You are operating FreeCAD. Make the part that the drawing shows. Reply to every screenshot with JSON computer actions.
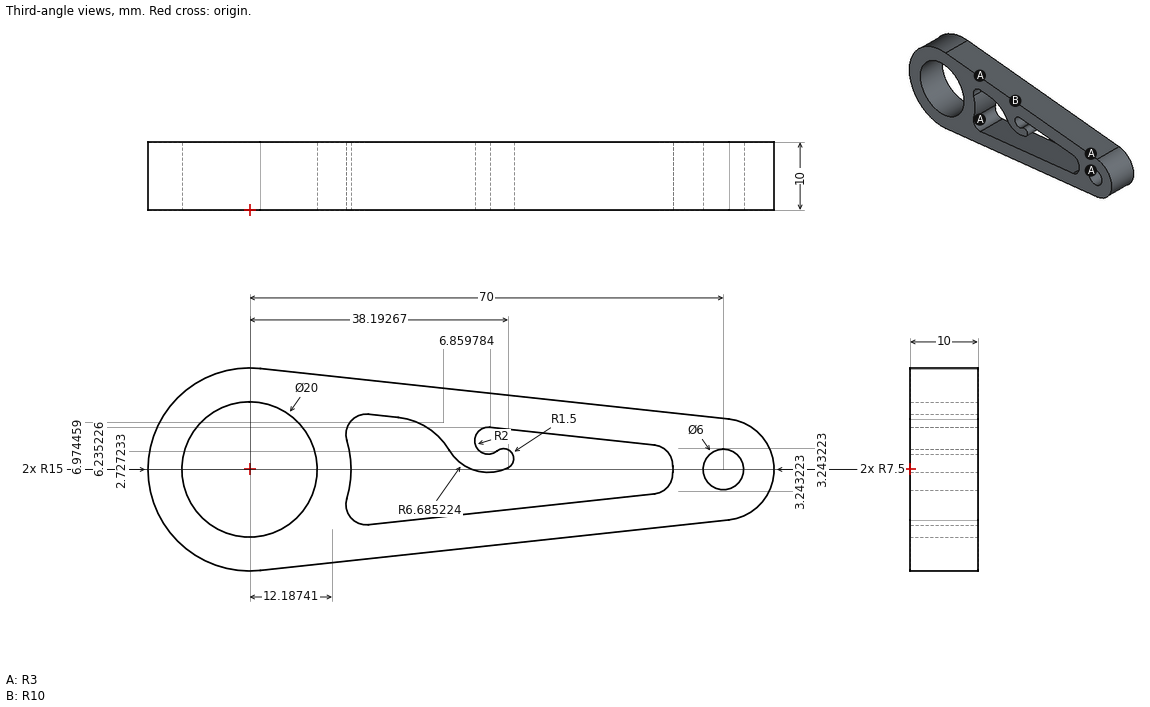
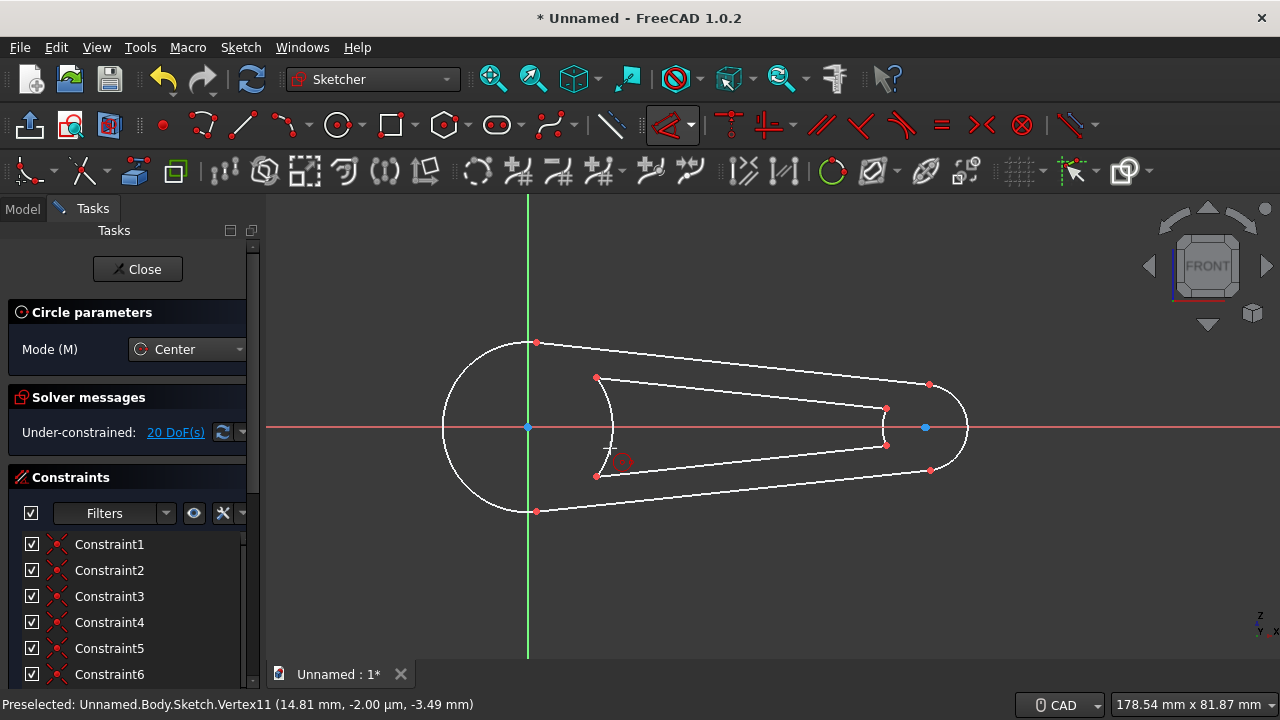
{"action": "scroll", "coordinate": [925, 427], "scroll_direction": "up", "scroll_amount": 2}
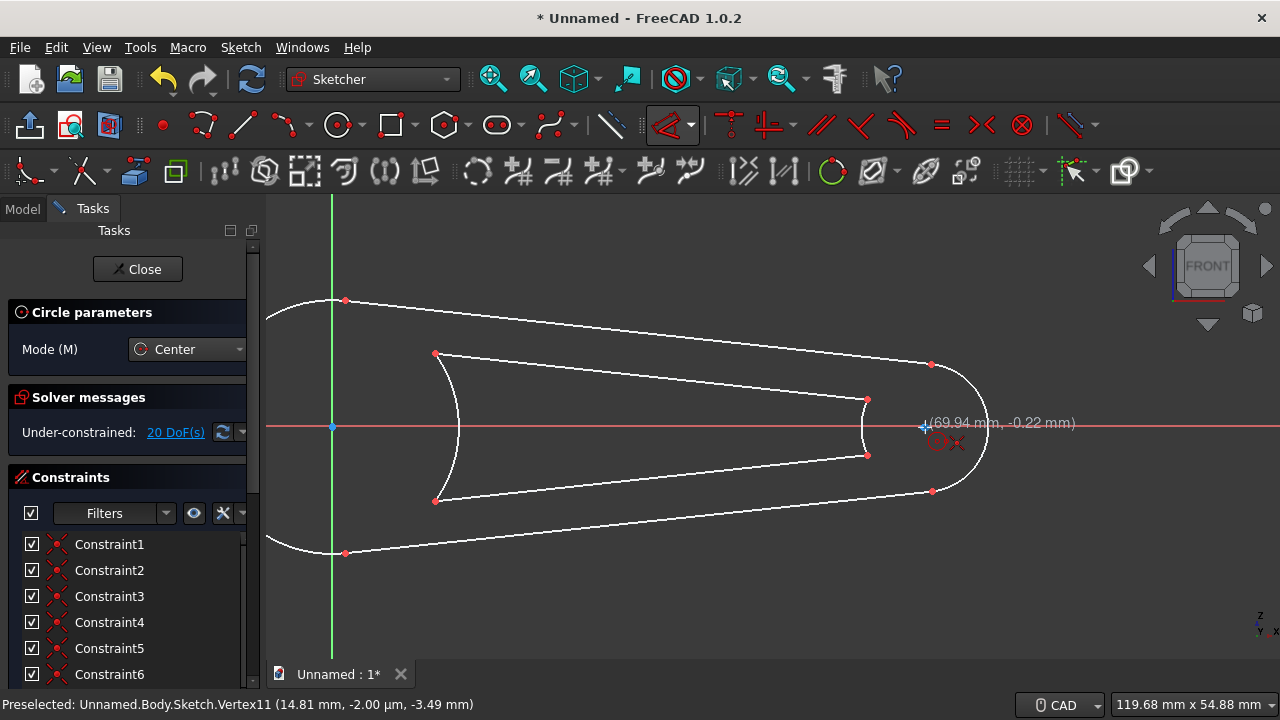
{"action": "left_click", "coordinate": [925, 426]}
{"action": "mouse_move", "coordinate": [943, 408]}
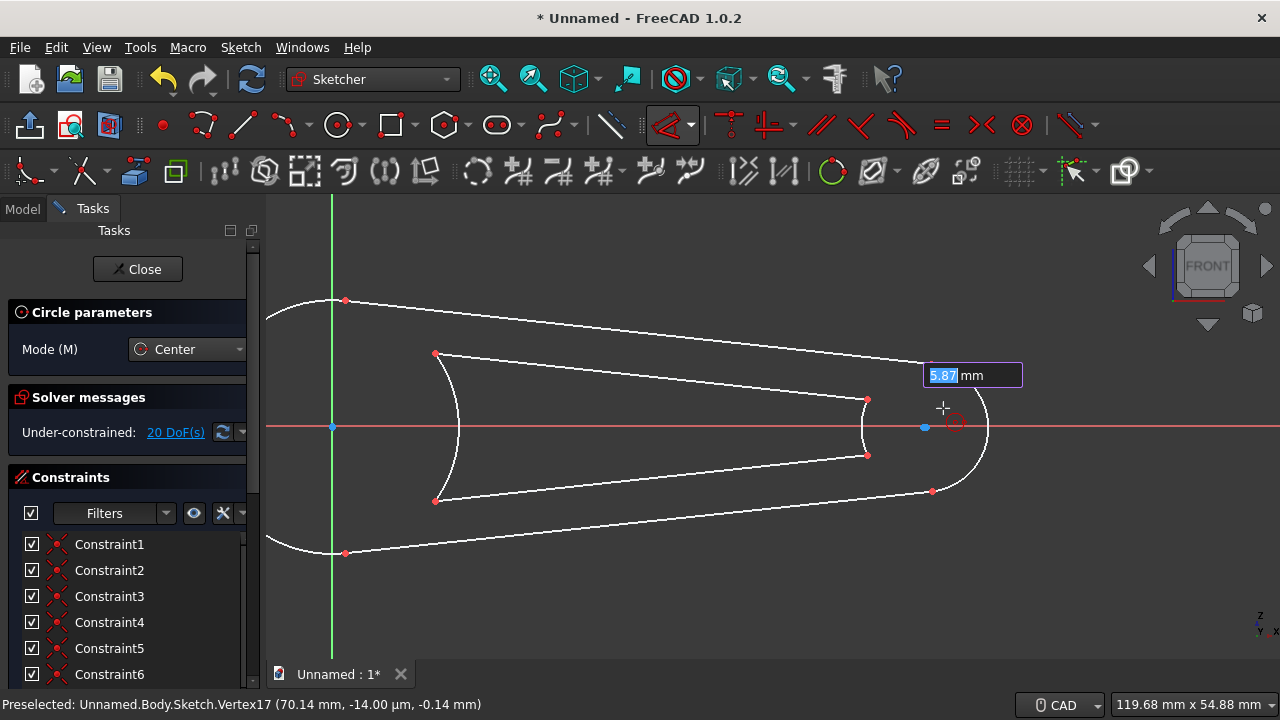
{"action": "type", "text": "6"}
{"action": "key", "text": "Return"}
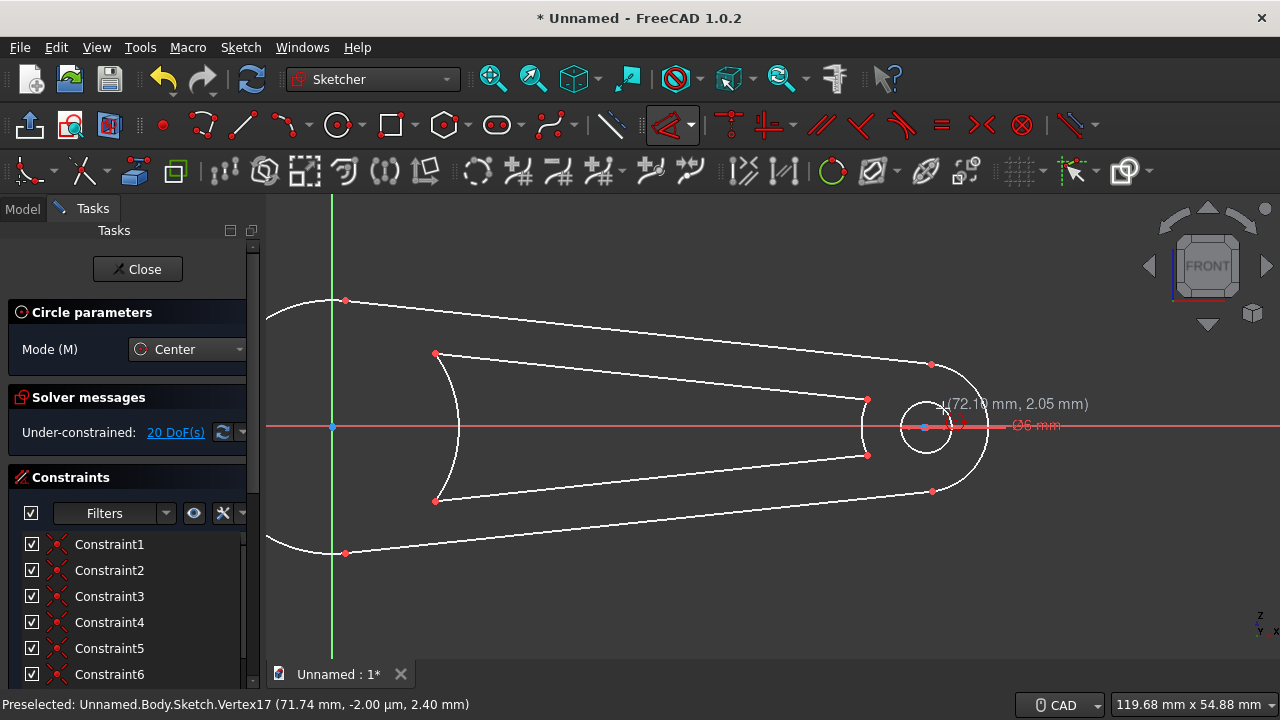
{"action": "left_click", "coordinate": [332, 426]}
{"action": "mouse_move", "coordinate": [392, 366]}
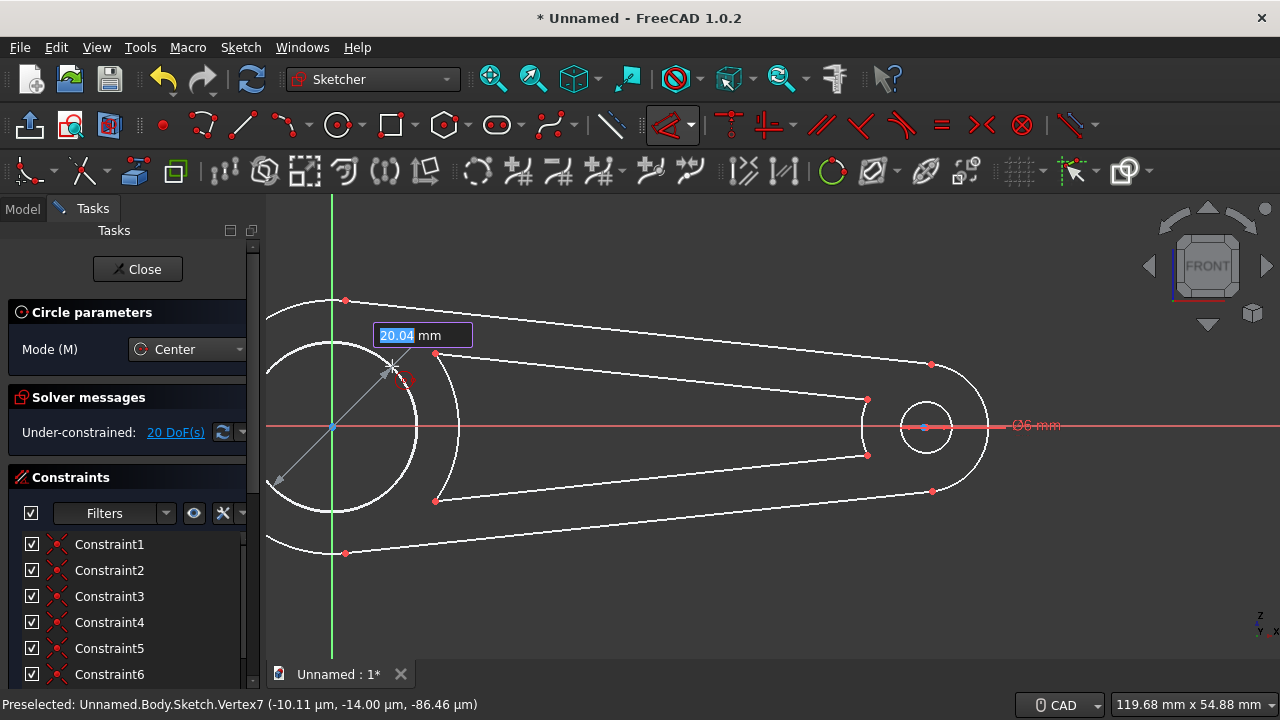
{"action": "type", "text": "20"}
{"action": "key", "text": "Return"}
{"action": "key", "text": "Escape"}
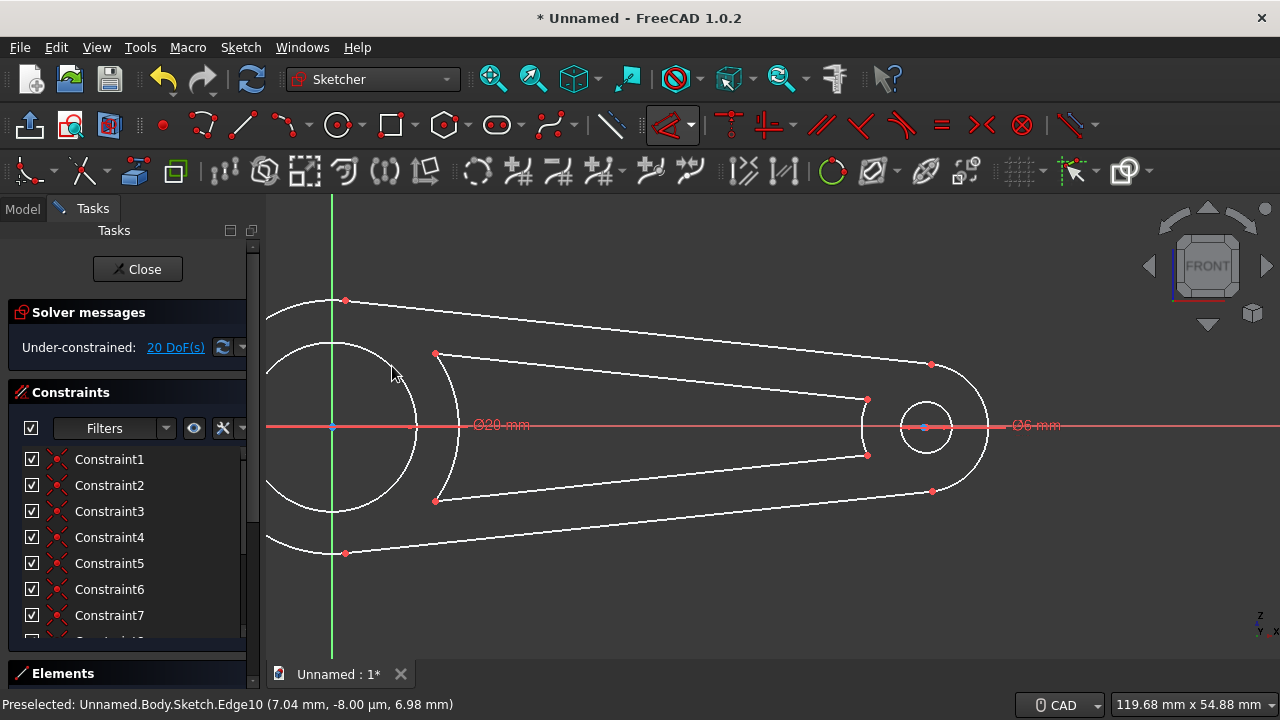
{"action": "left_click", "coordinate": [756, 510]}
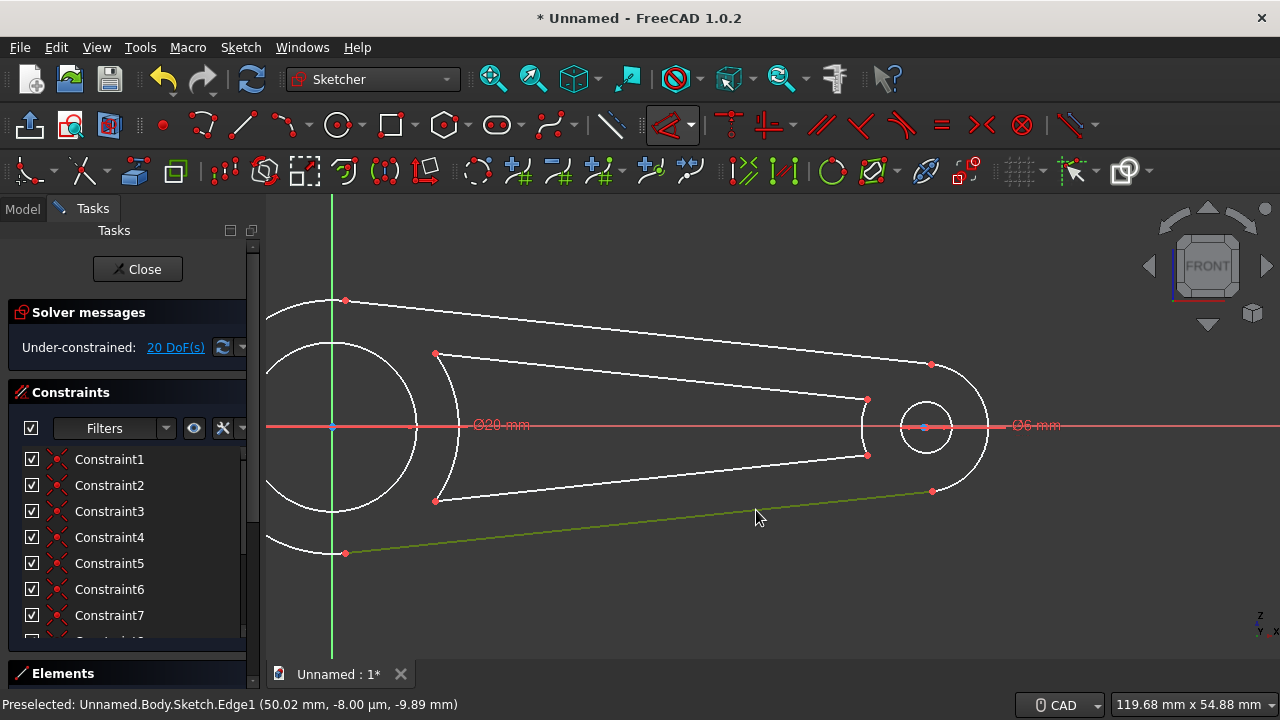
{"action": "scroll", "coordinate": [923, 427], "scroll_direction": "down", "scroll_amount": 2}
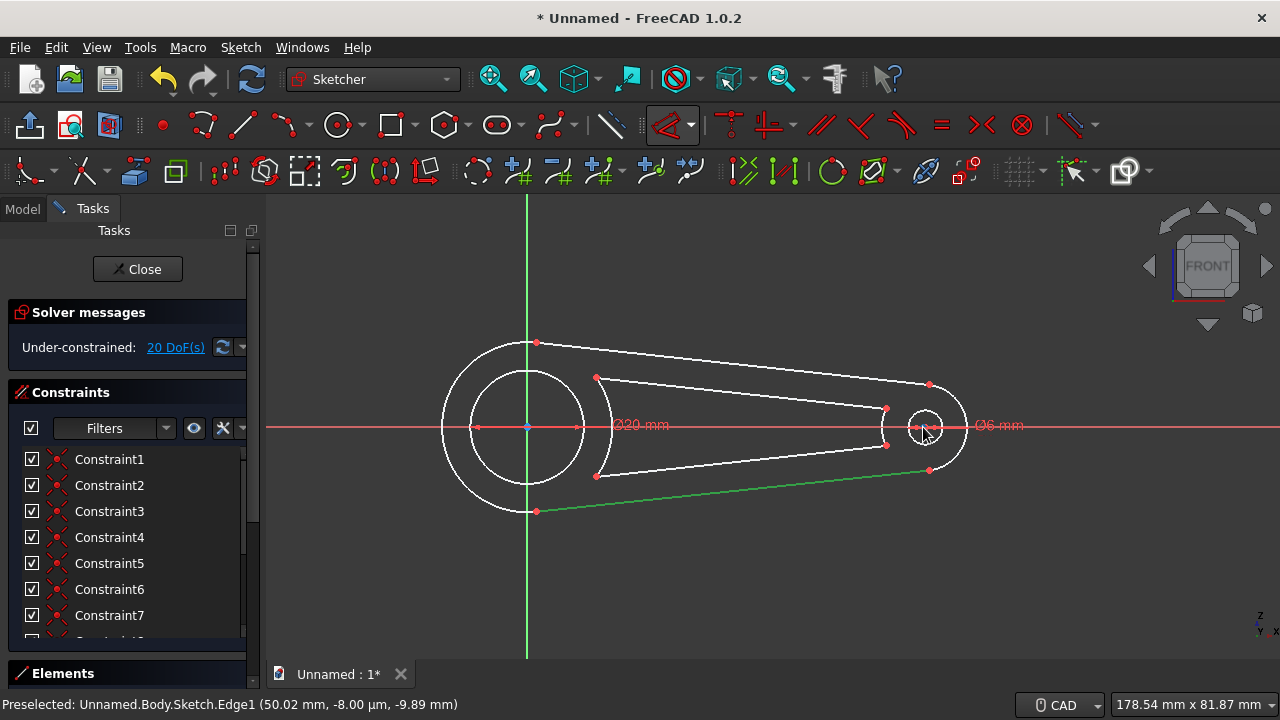
{"action": "left_click", "coordinate": [461, 374]}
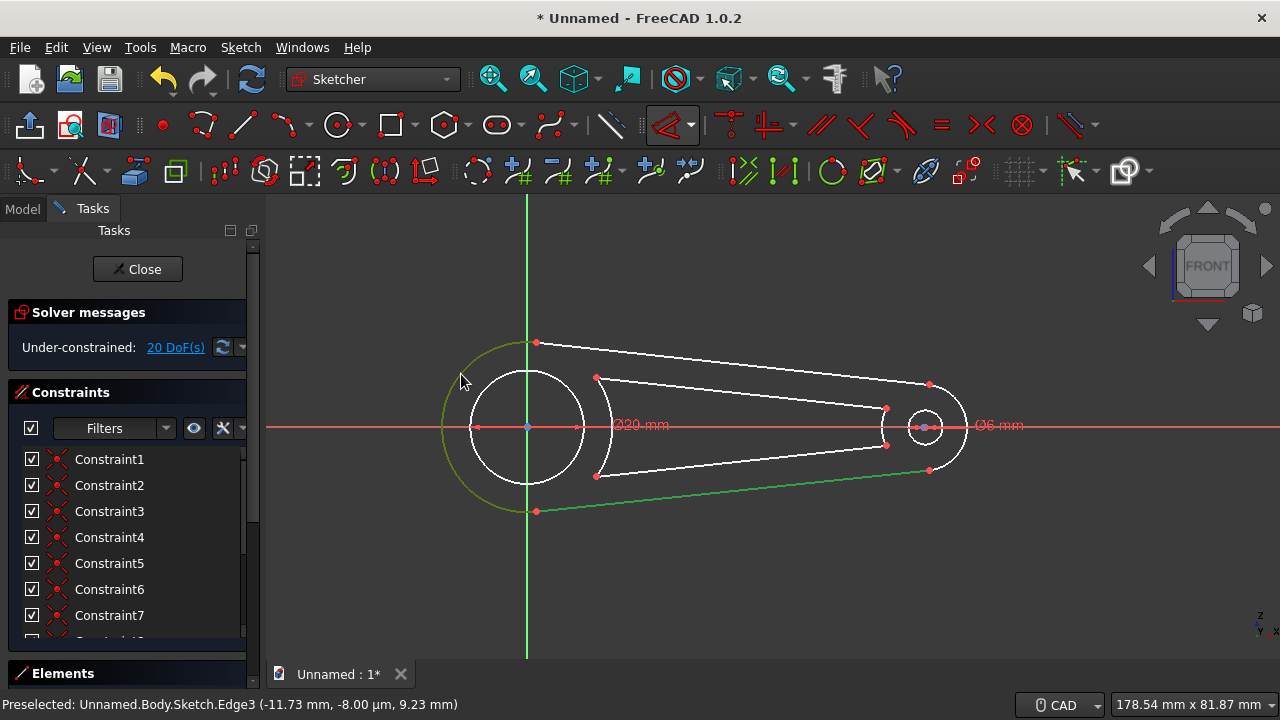
{"action": "left_click", "coordinate": [902, 126]}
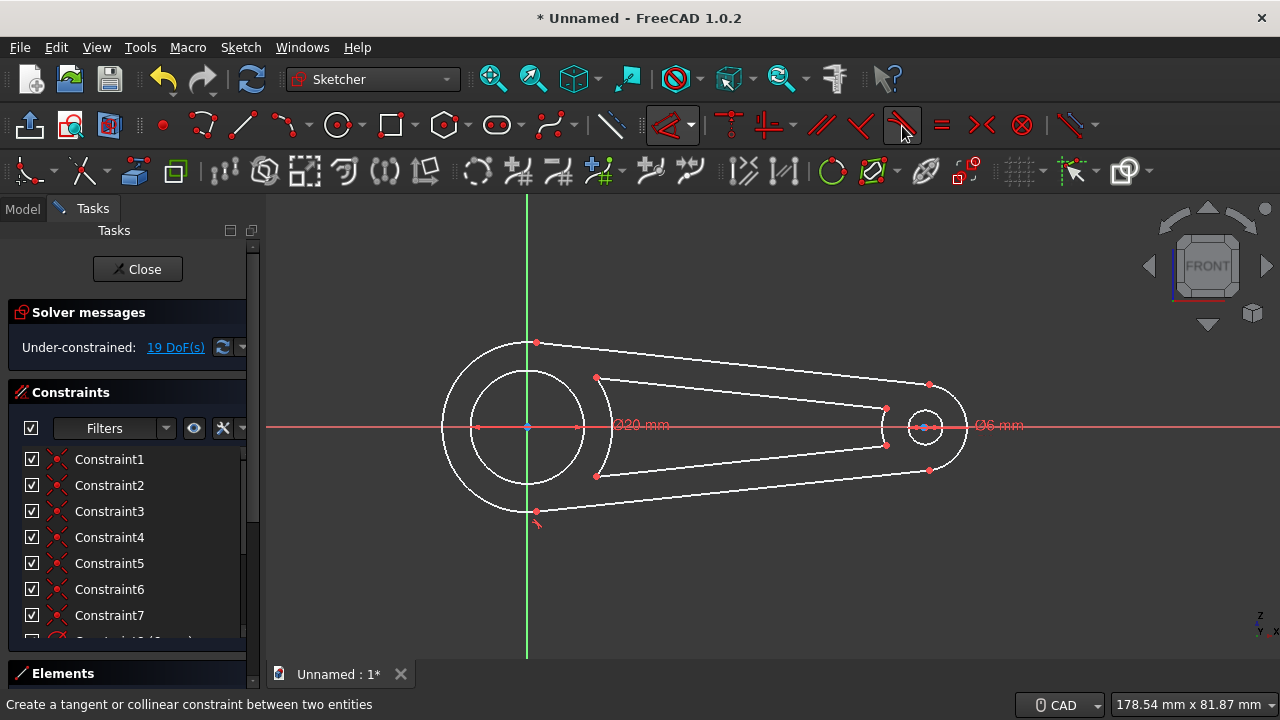
{"action": "left_click", "coordinate": [812, 483]}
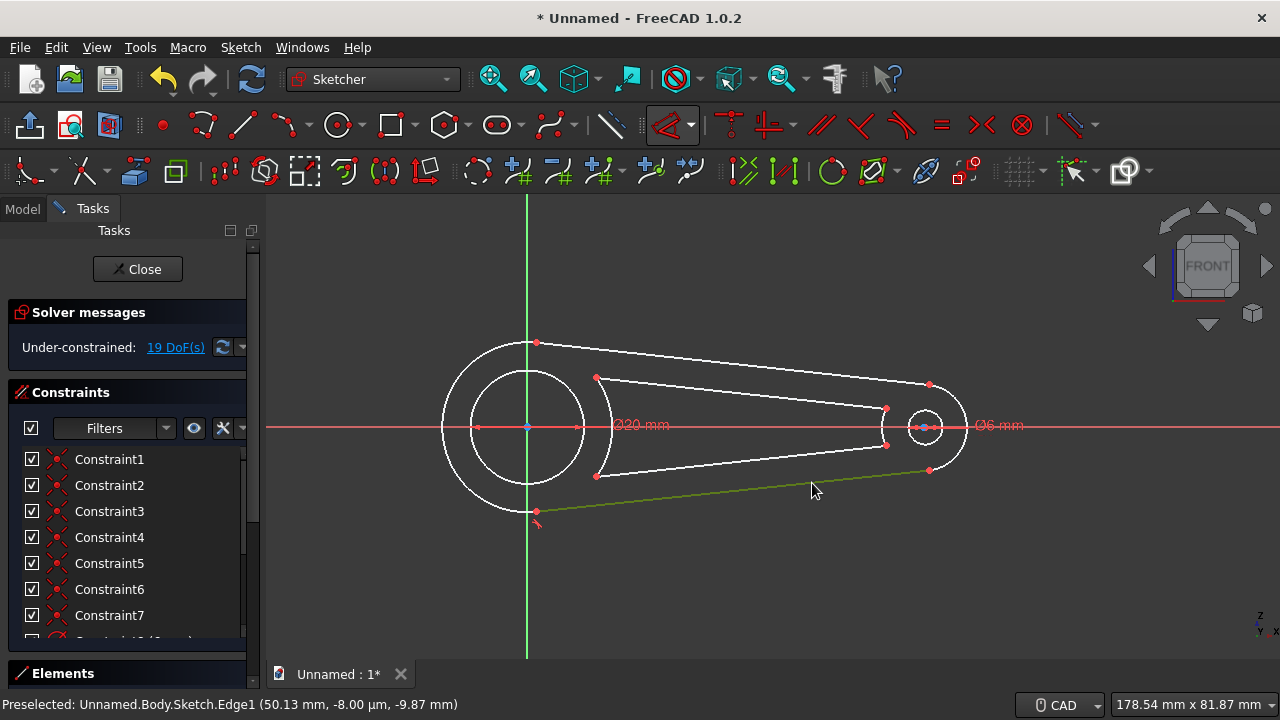
{"action": "left_click", "coordinate": [960, 451]}